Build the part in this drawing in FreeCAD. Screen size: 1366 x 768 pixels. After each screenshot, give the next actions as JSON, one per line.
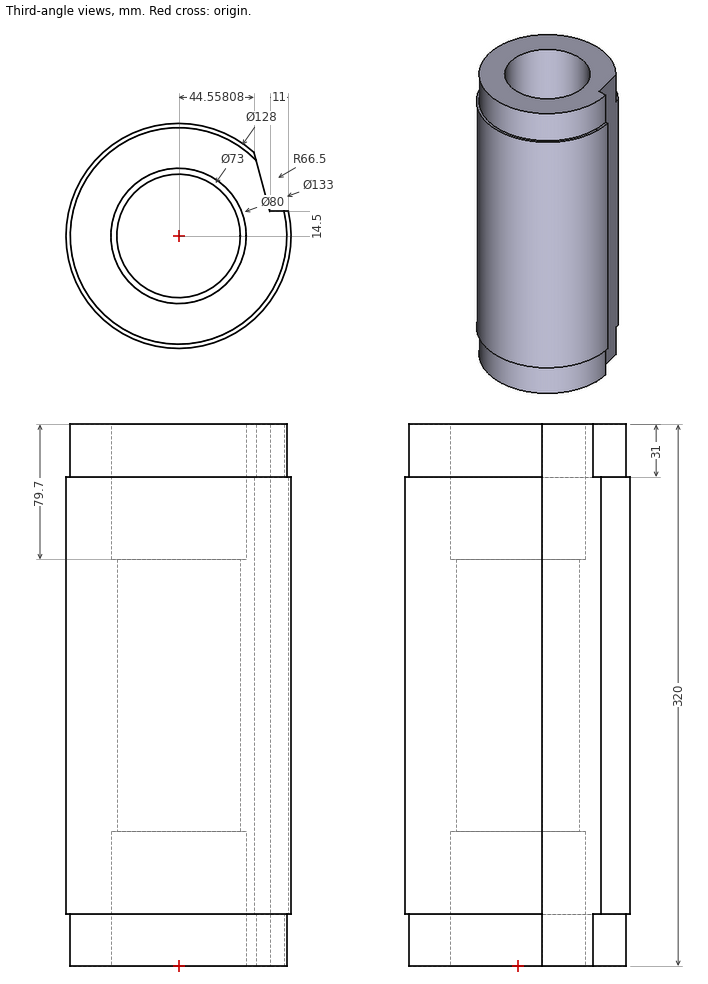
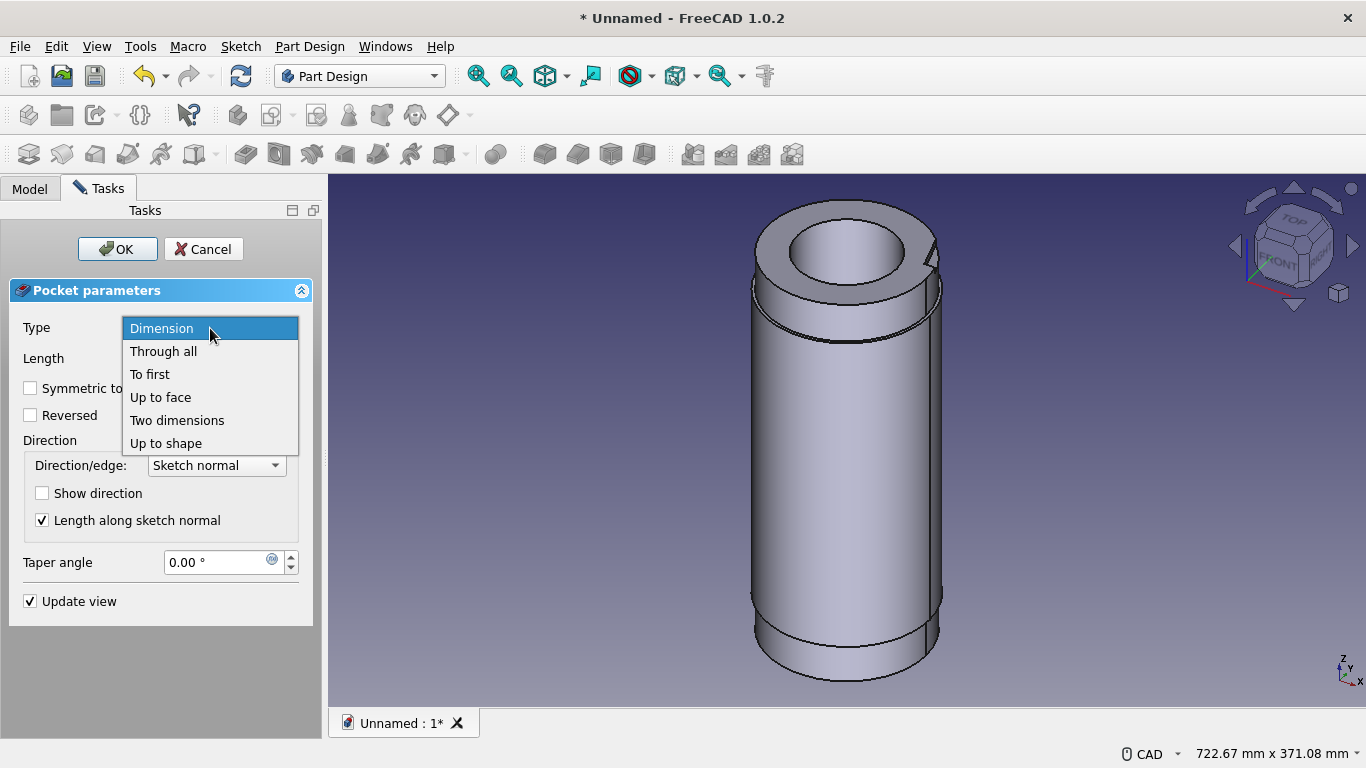
{"action": "left_click", "coordinate": [208, 352]}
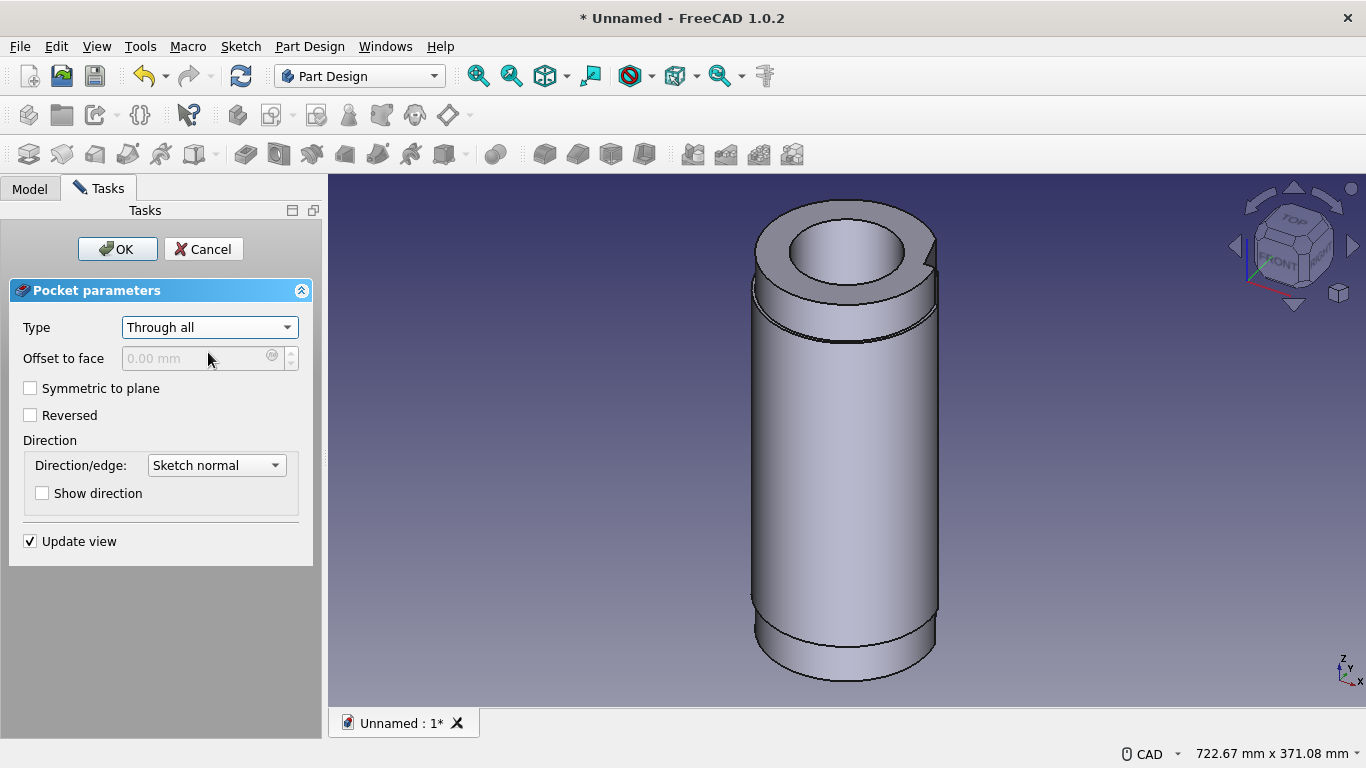
{"action": "left_click", "coordinate": [118, 249]}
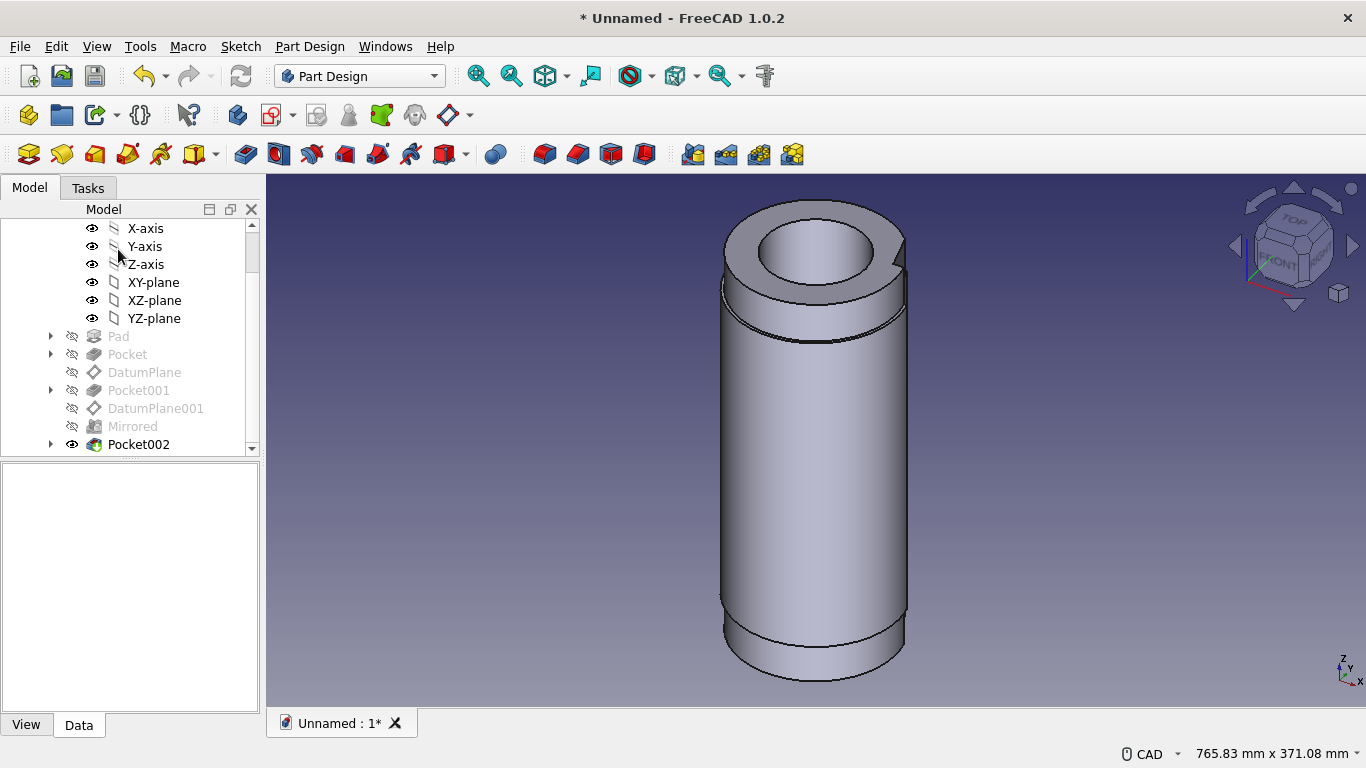
{"action": "key", "text": "0"}